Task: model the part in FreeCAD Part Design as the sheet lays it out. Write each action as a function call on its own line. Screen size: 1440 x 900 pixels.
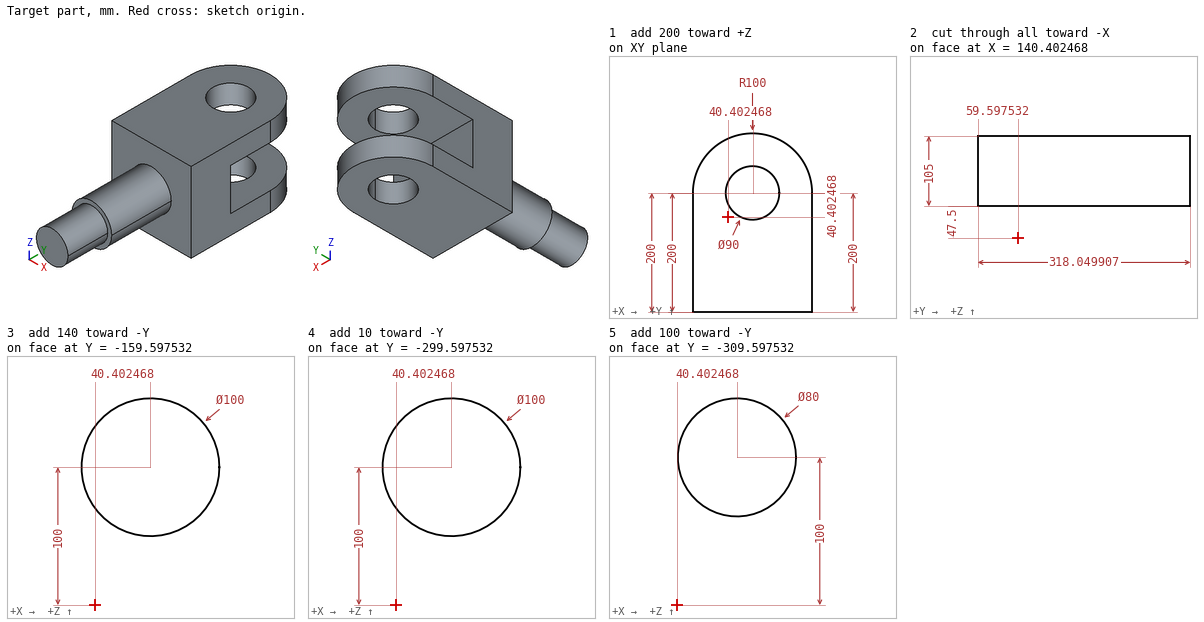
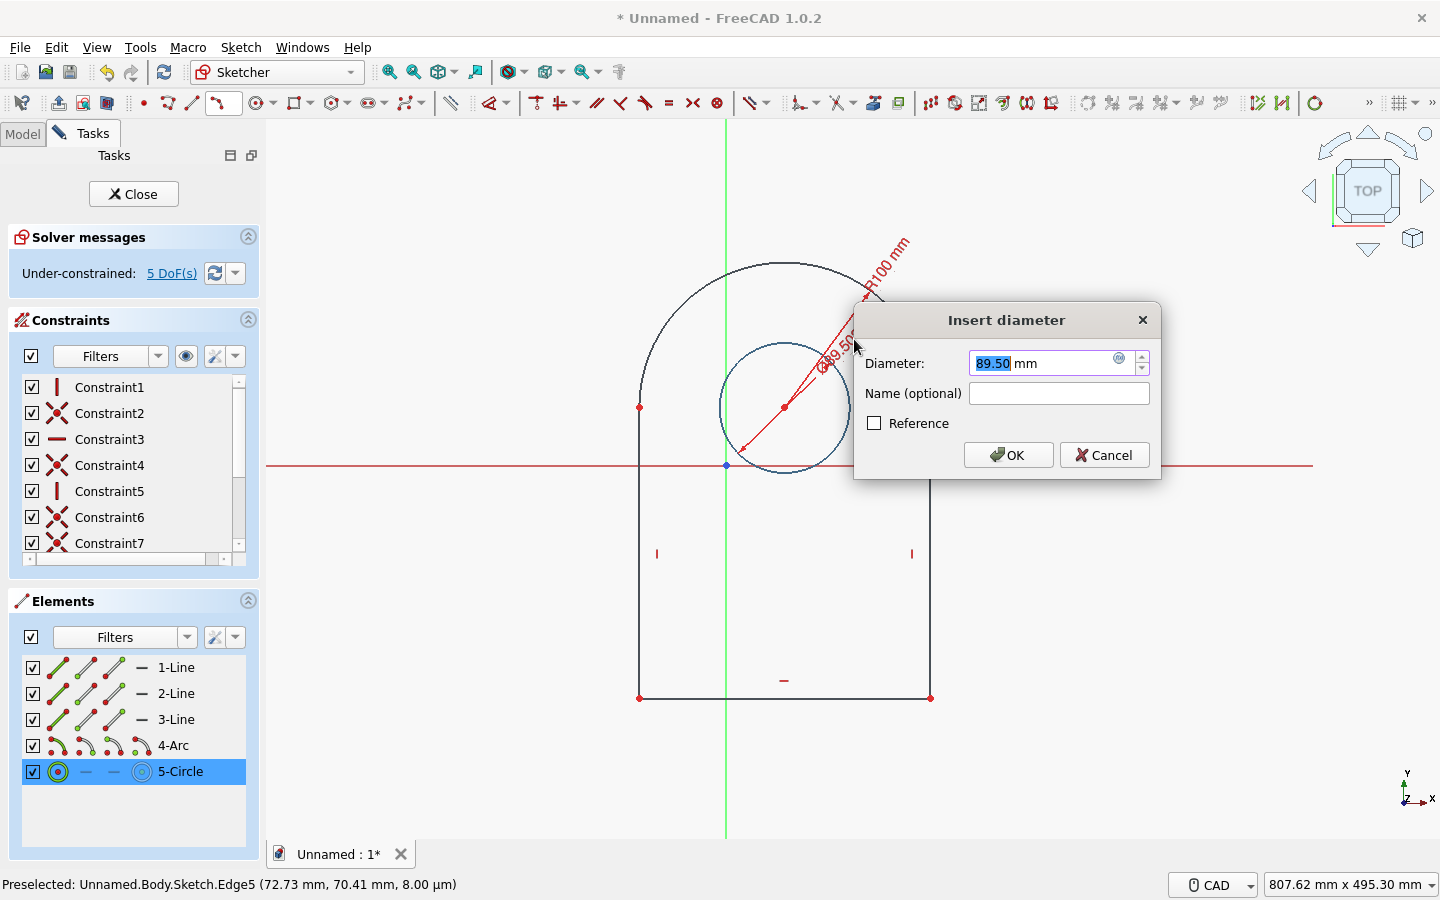
text(90)
key(Return)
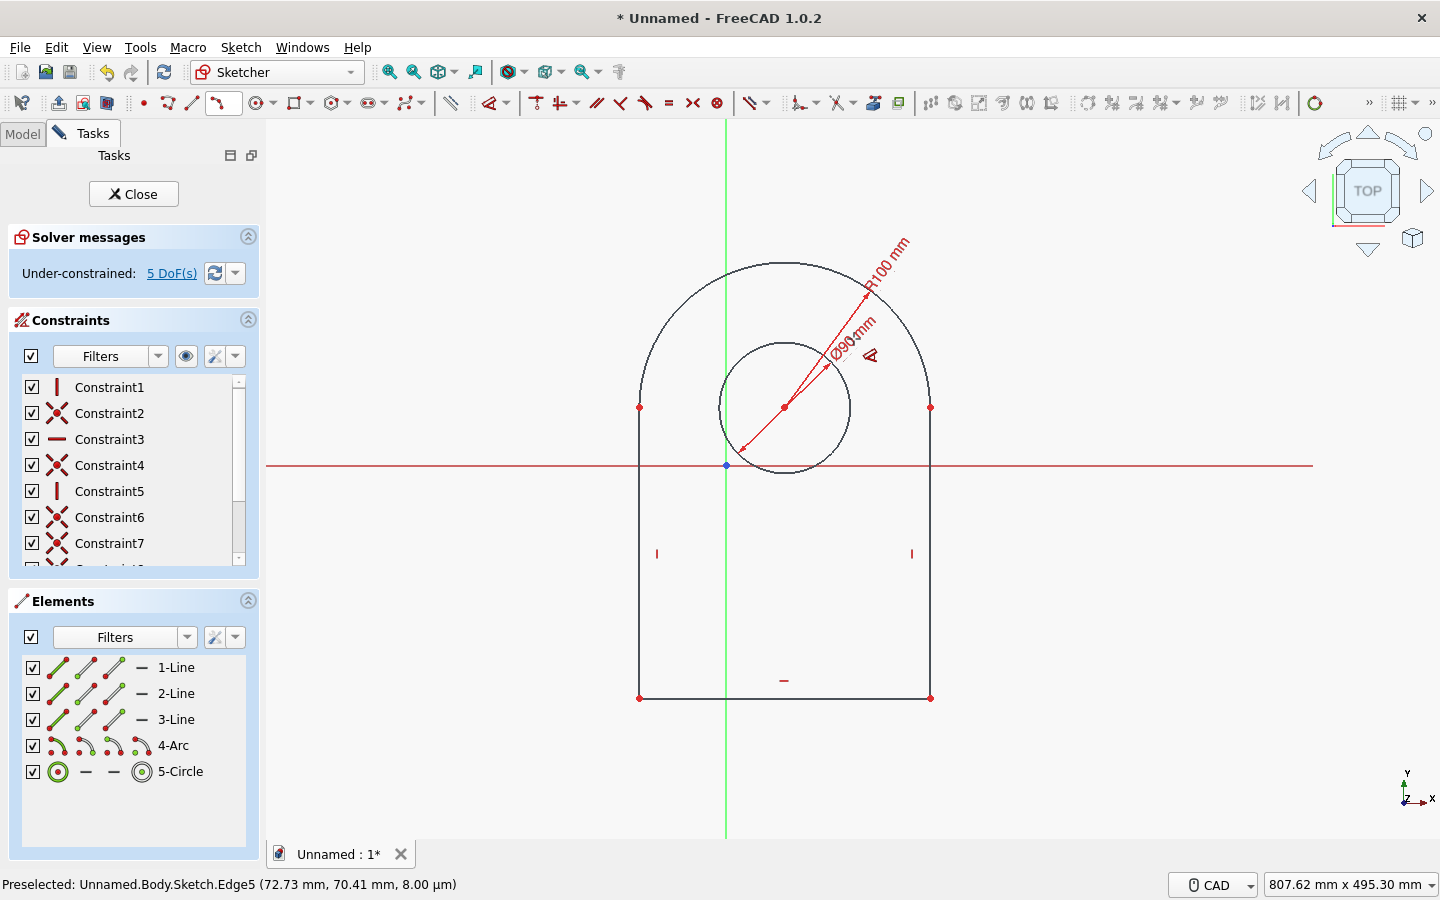
click(639, 495)
click(605, 553)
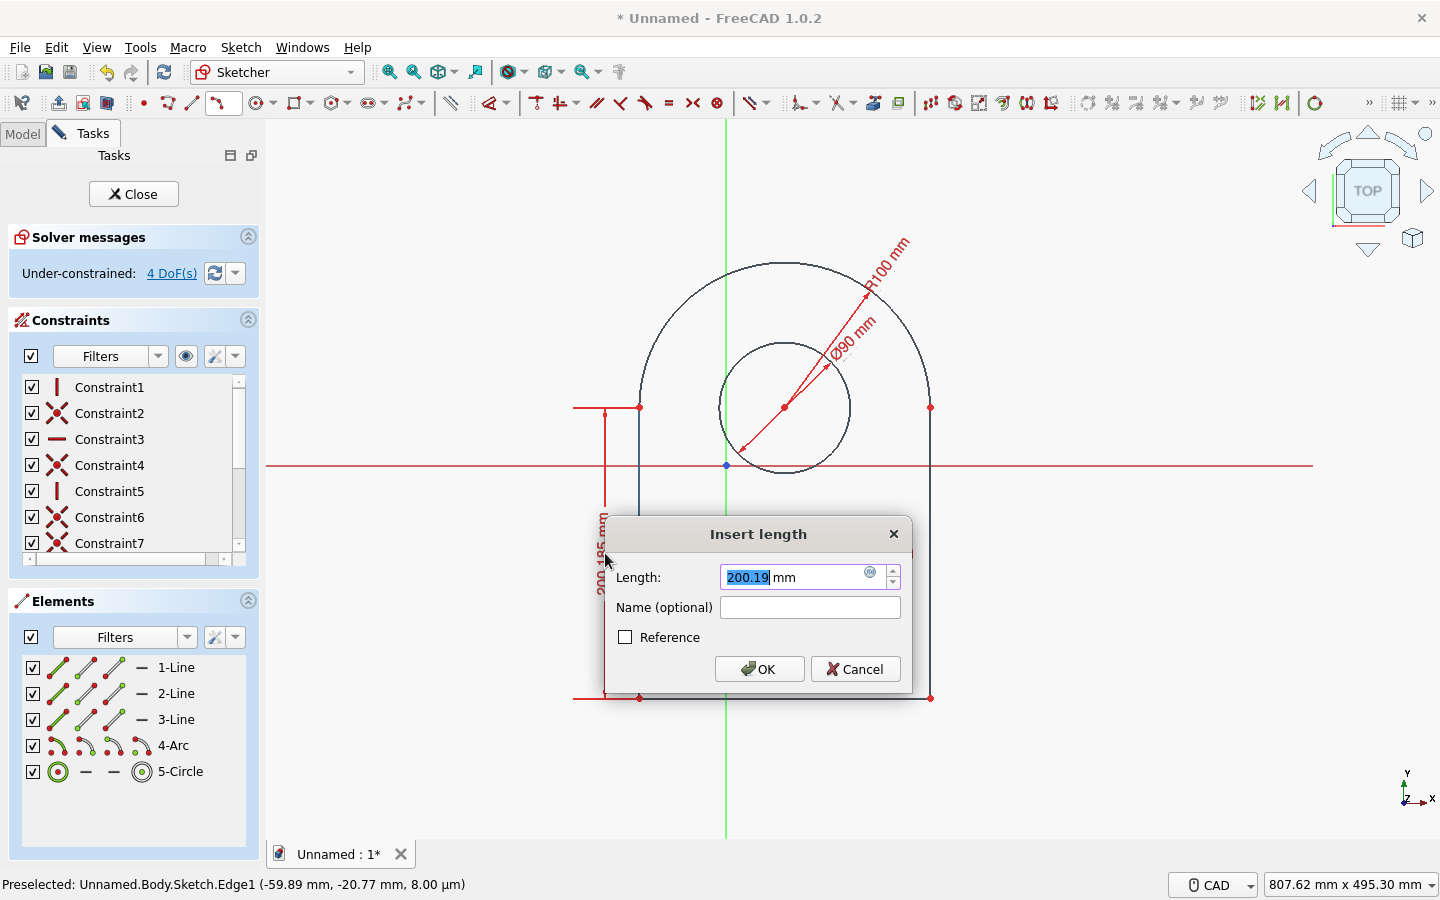
text(200)
key(Return)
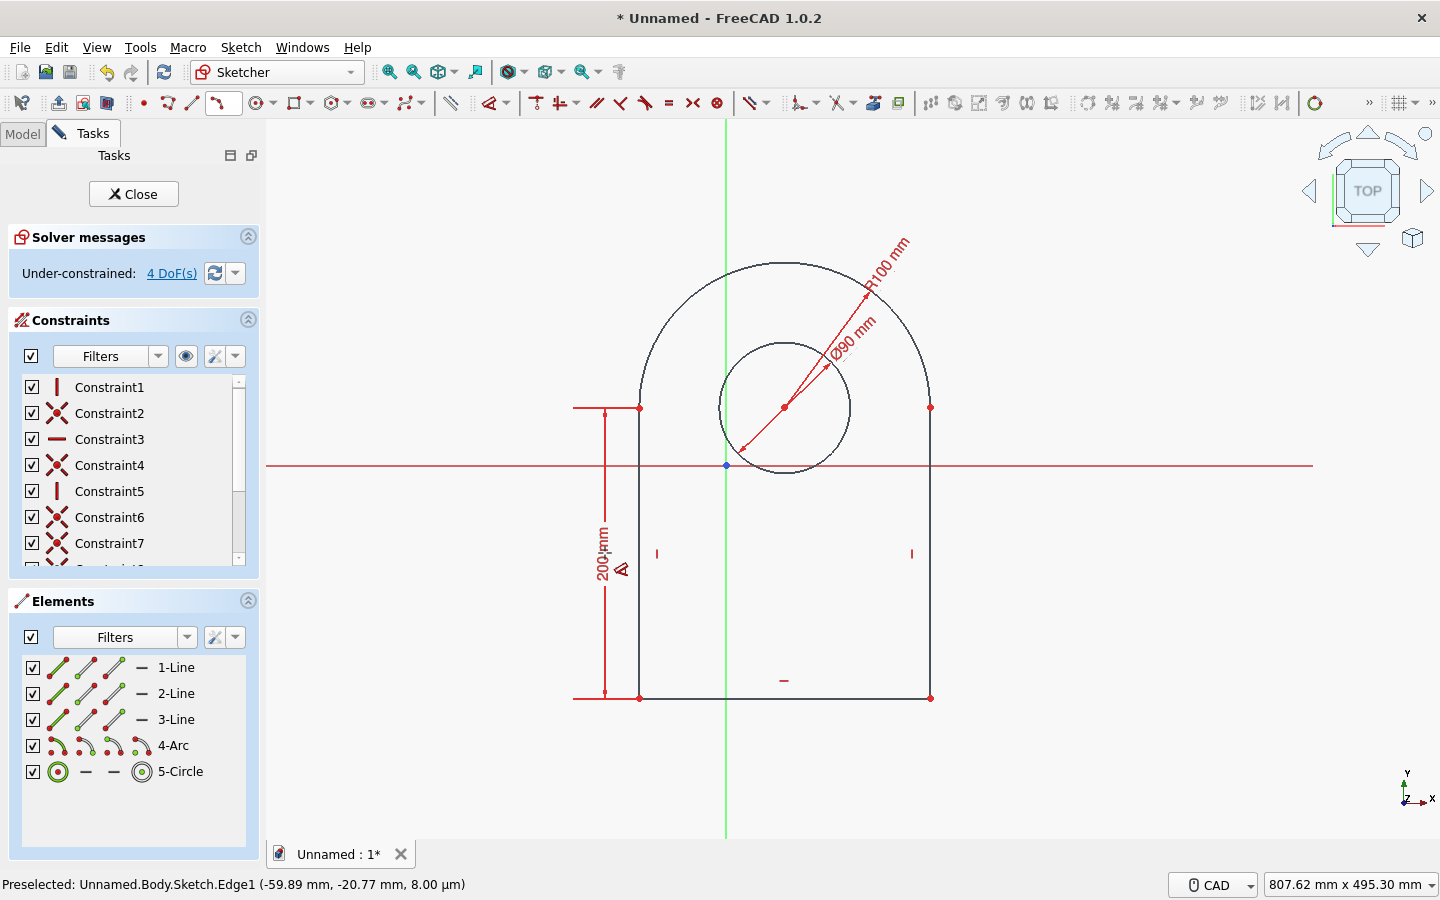
click(930, 612)
click(964, 553)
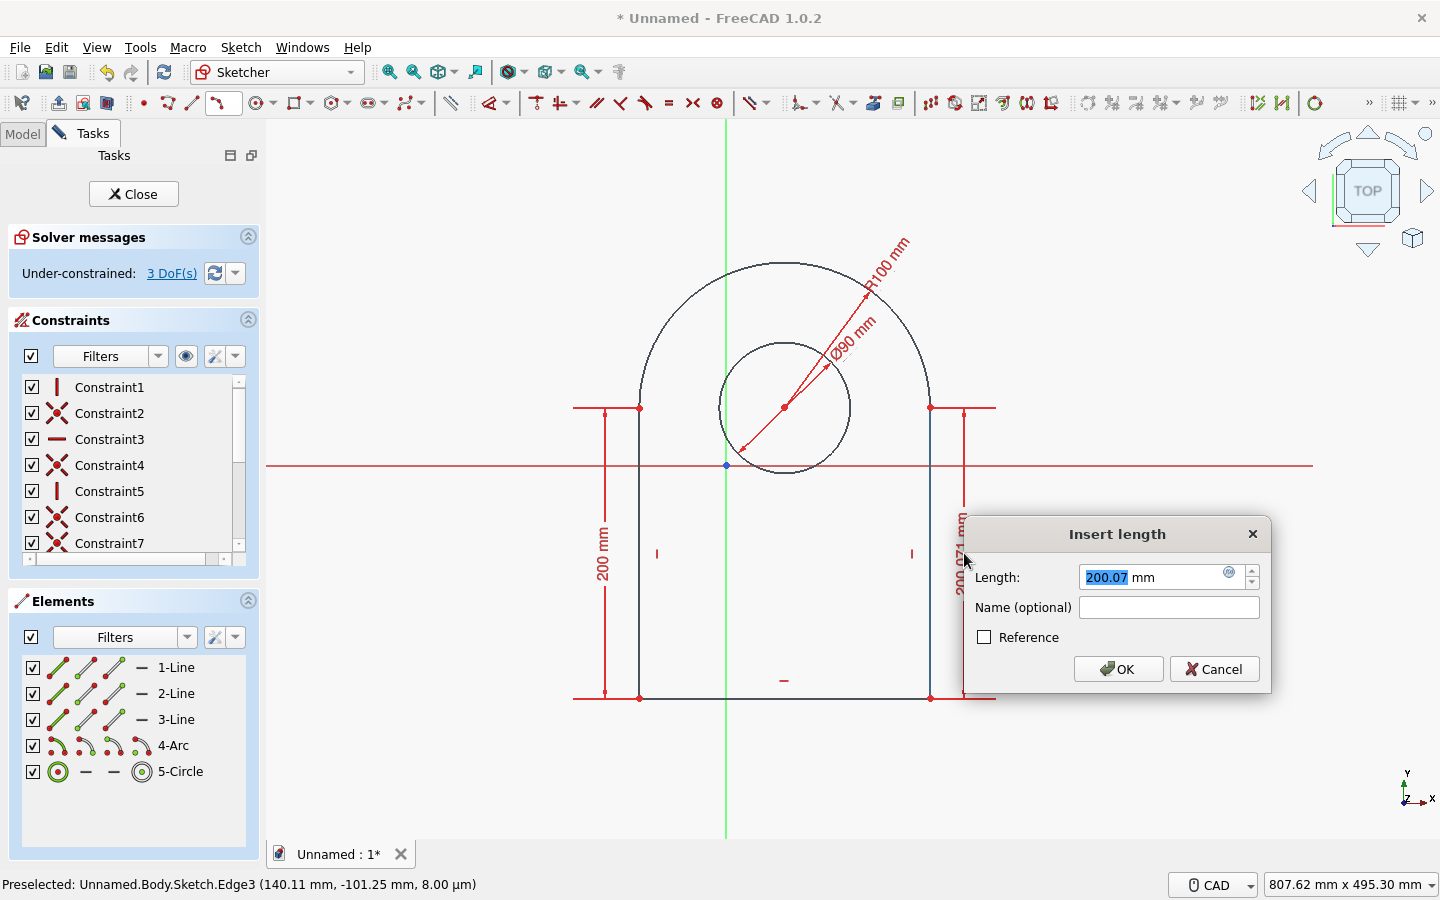
text(200)
key(Return)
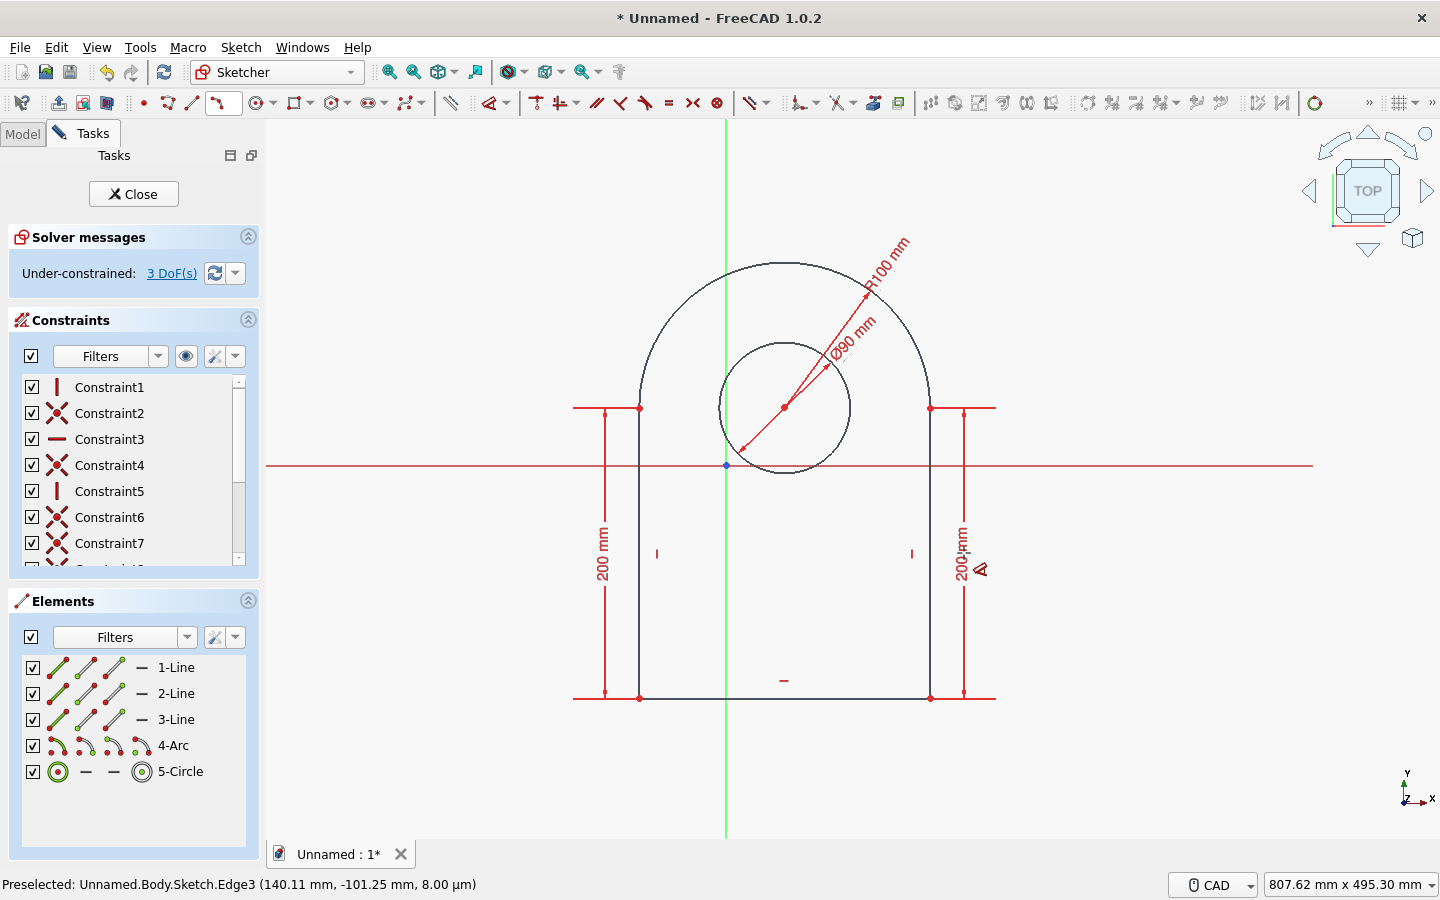
click(639, 699)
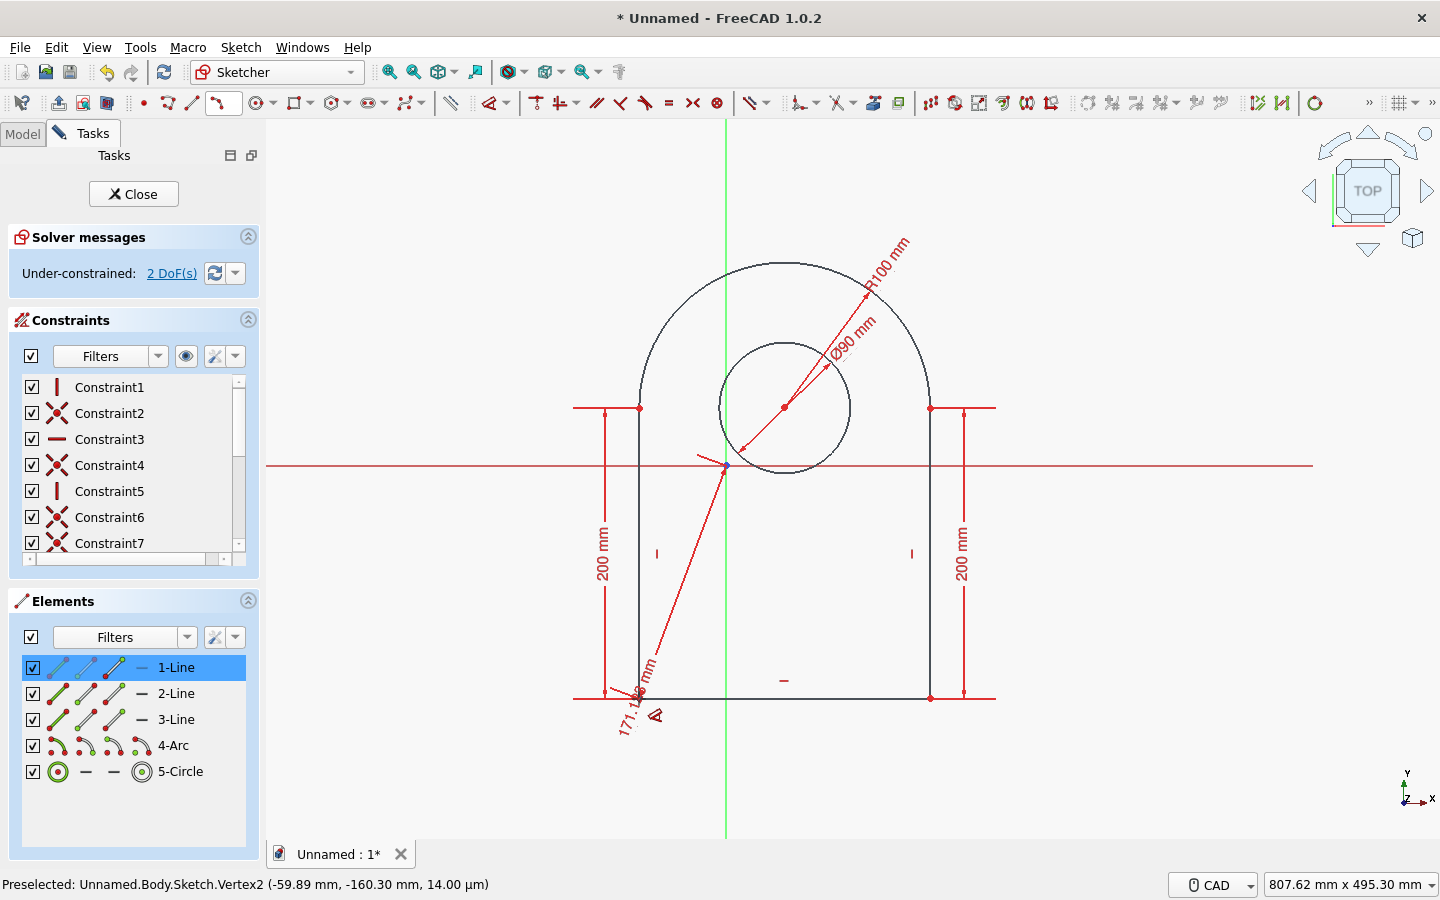
click(785, 408)
click(605, 487)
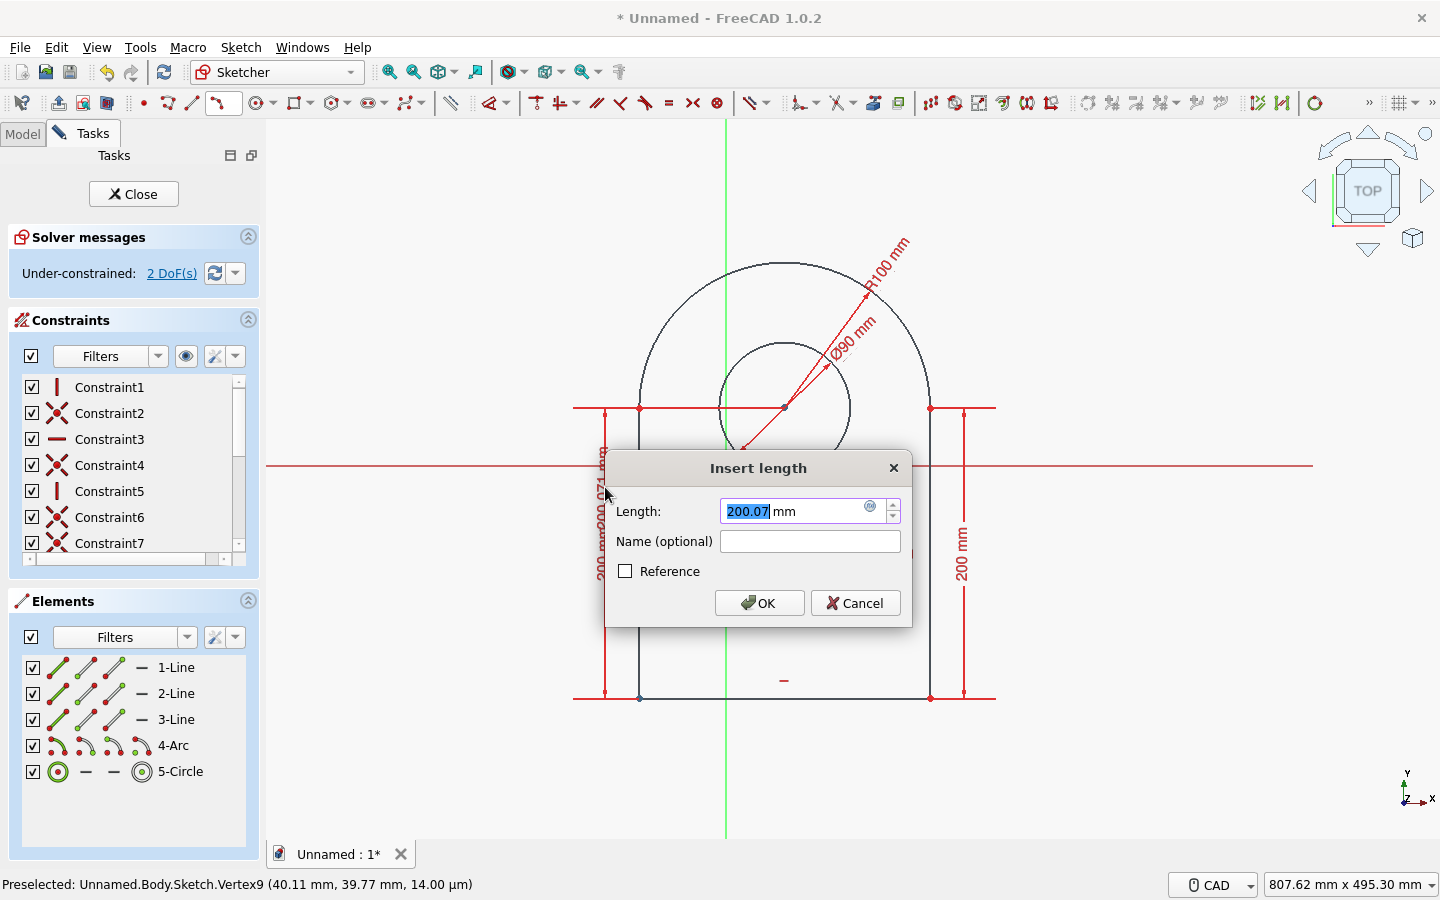
text(200)
key(Return)